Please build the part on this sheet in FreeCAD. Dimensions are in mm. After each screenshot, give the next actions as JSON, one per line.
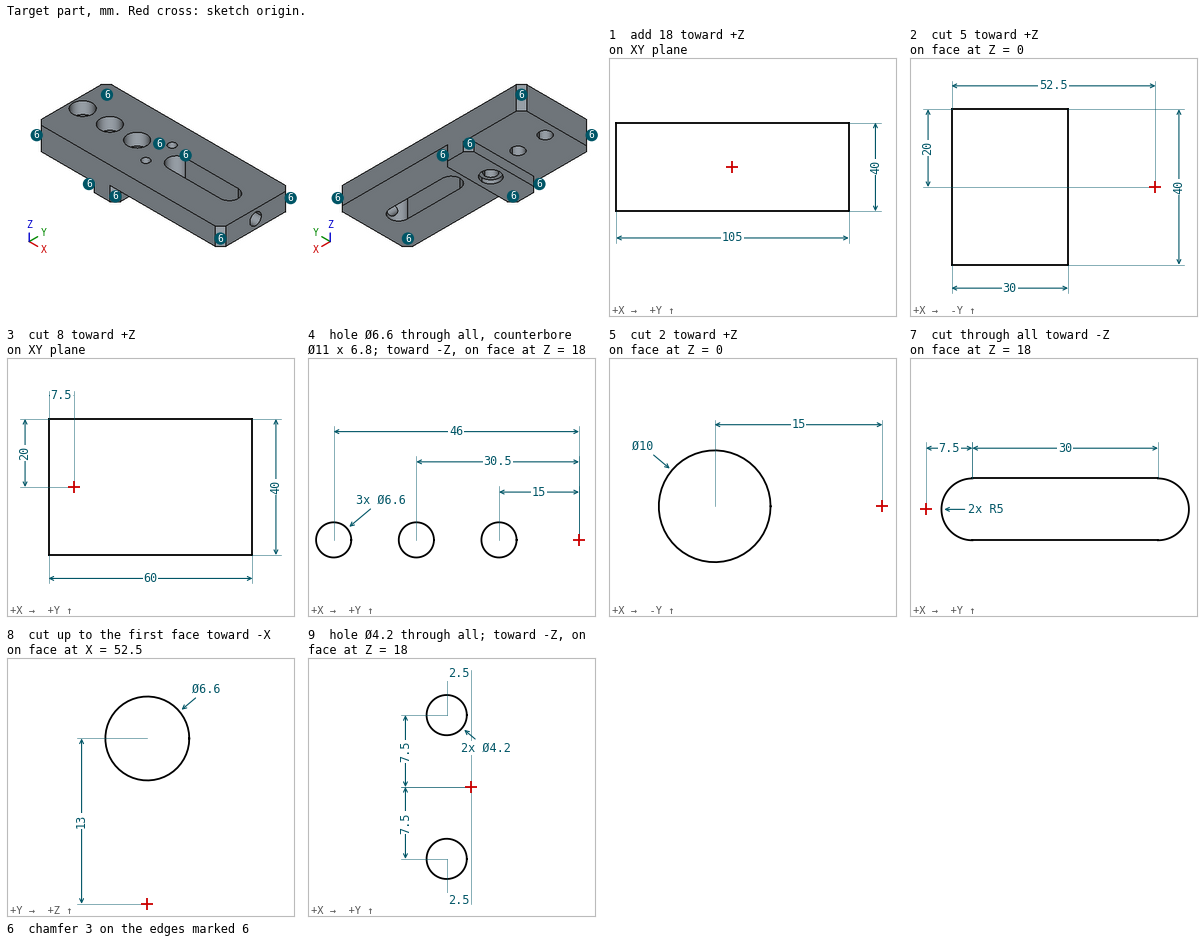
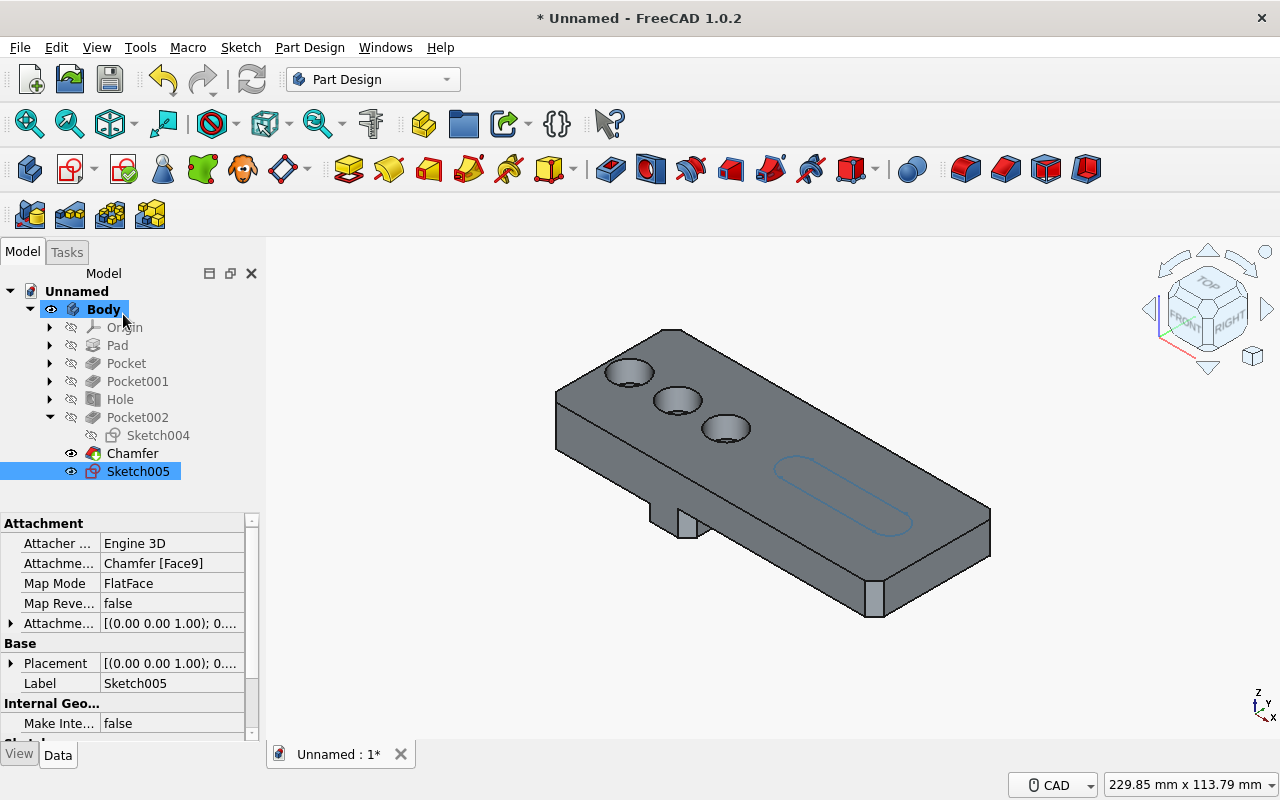
{"action": "left_click", "coordinate": [612, 170]}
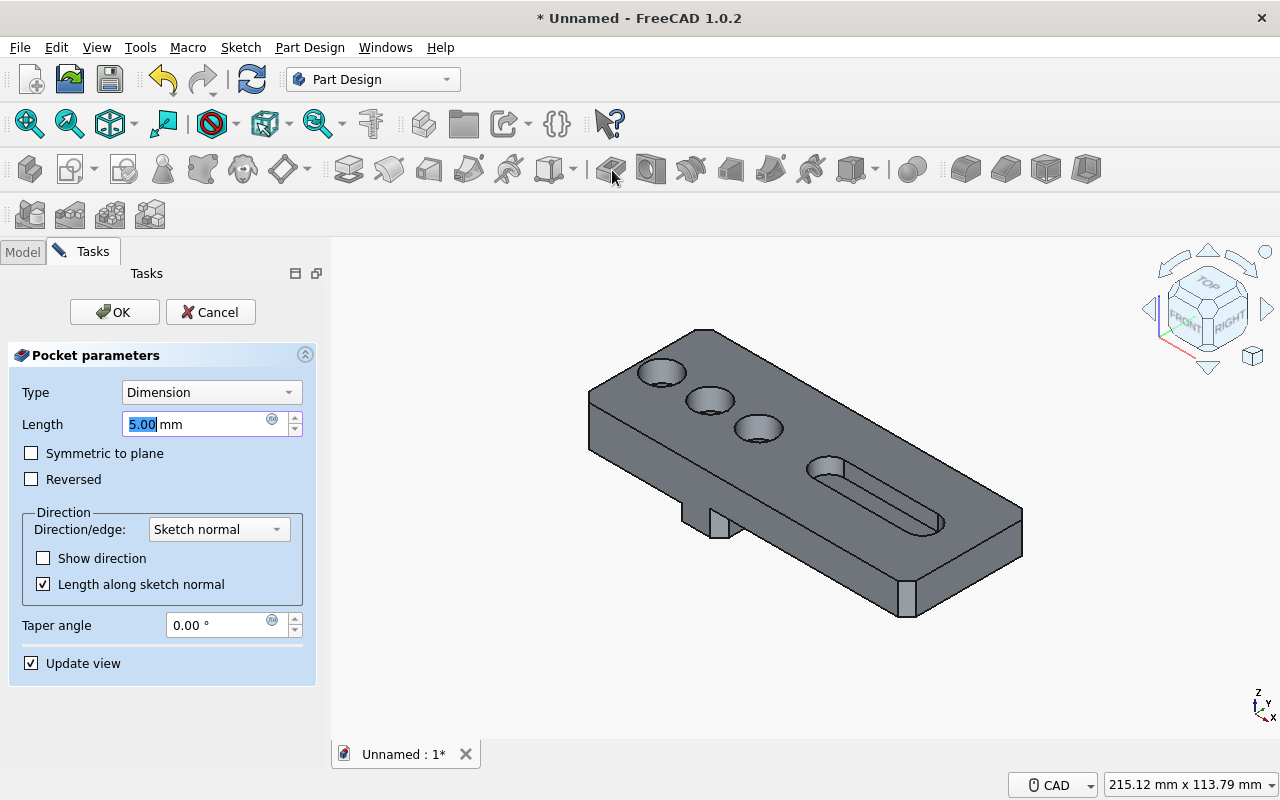
{"action": "left_click", "coordinate": [212, 392]}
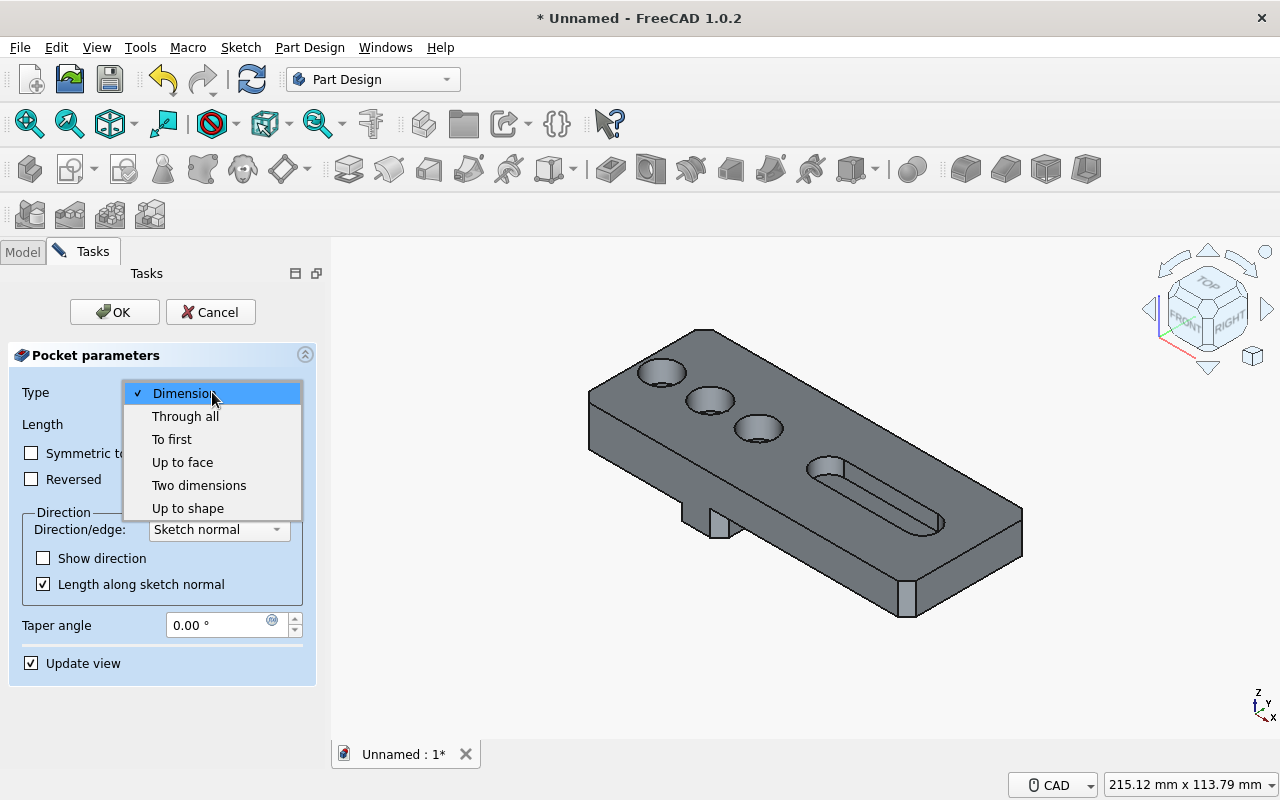
{"action": "left_click", "coordinate": [212, 416]}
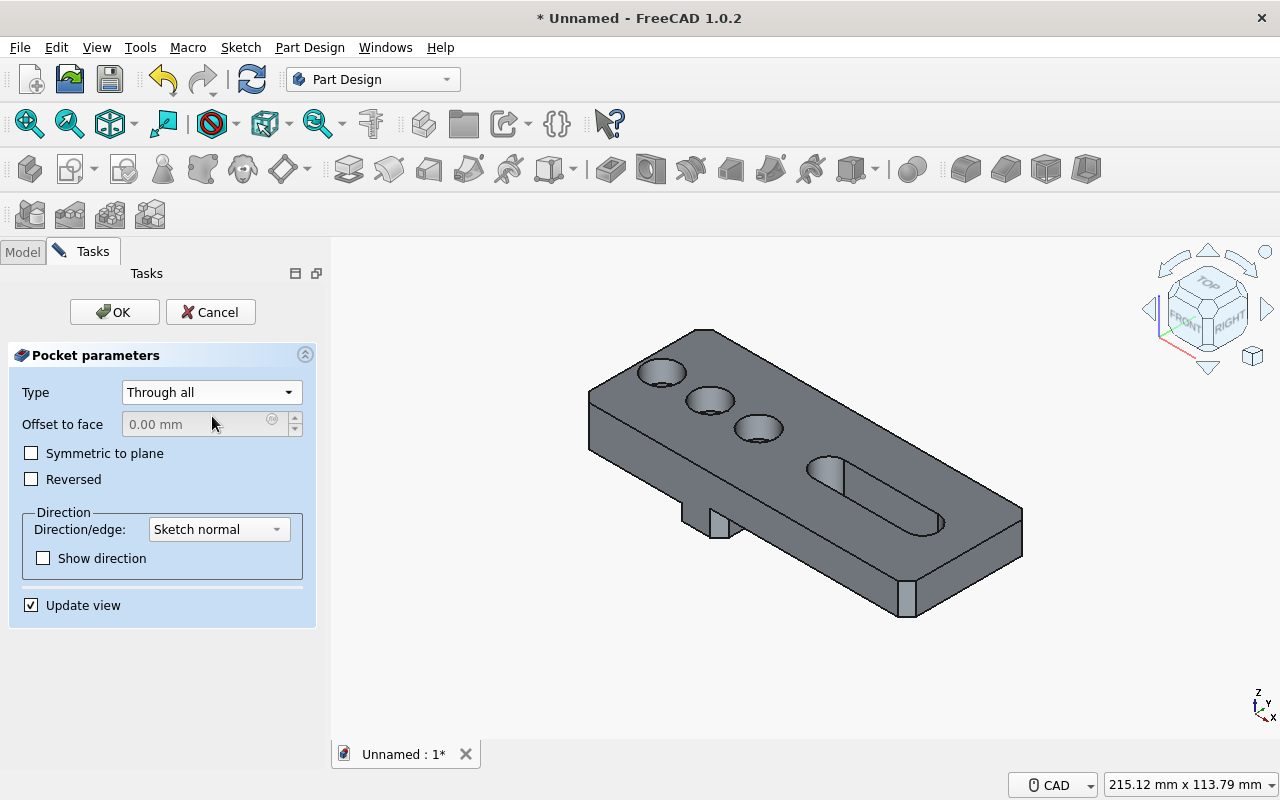
{"action": "left_click", "coordinate": [115, 312]}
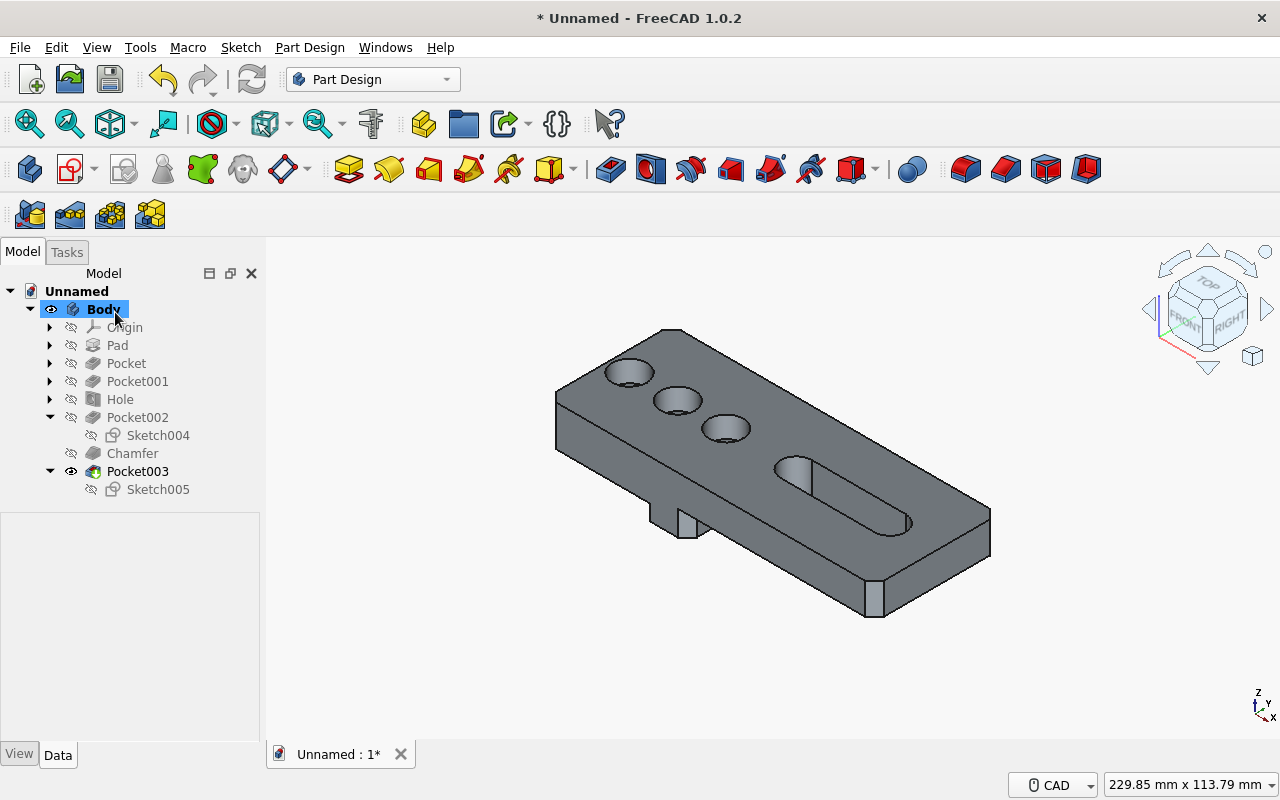
{"action": "left_click", "coordinate": [967, 550]}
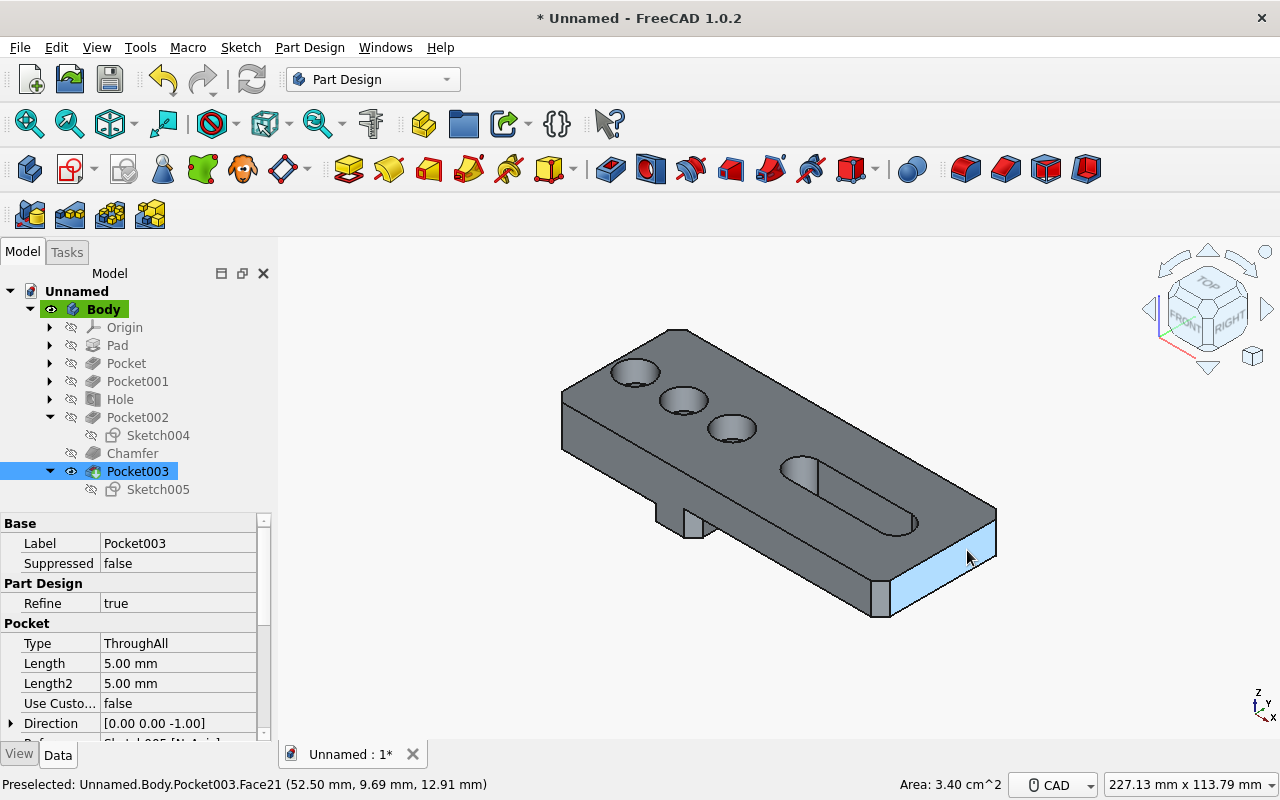
{"action": "left_click", "coordinate": [70, 170]}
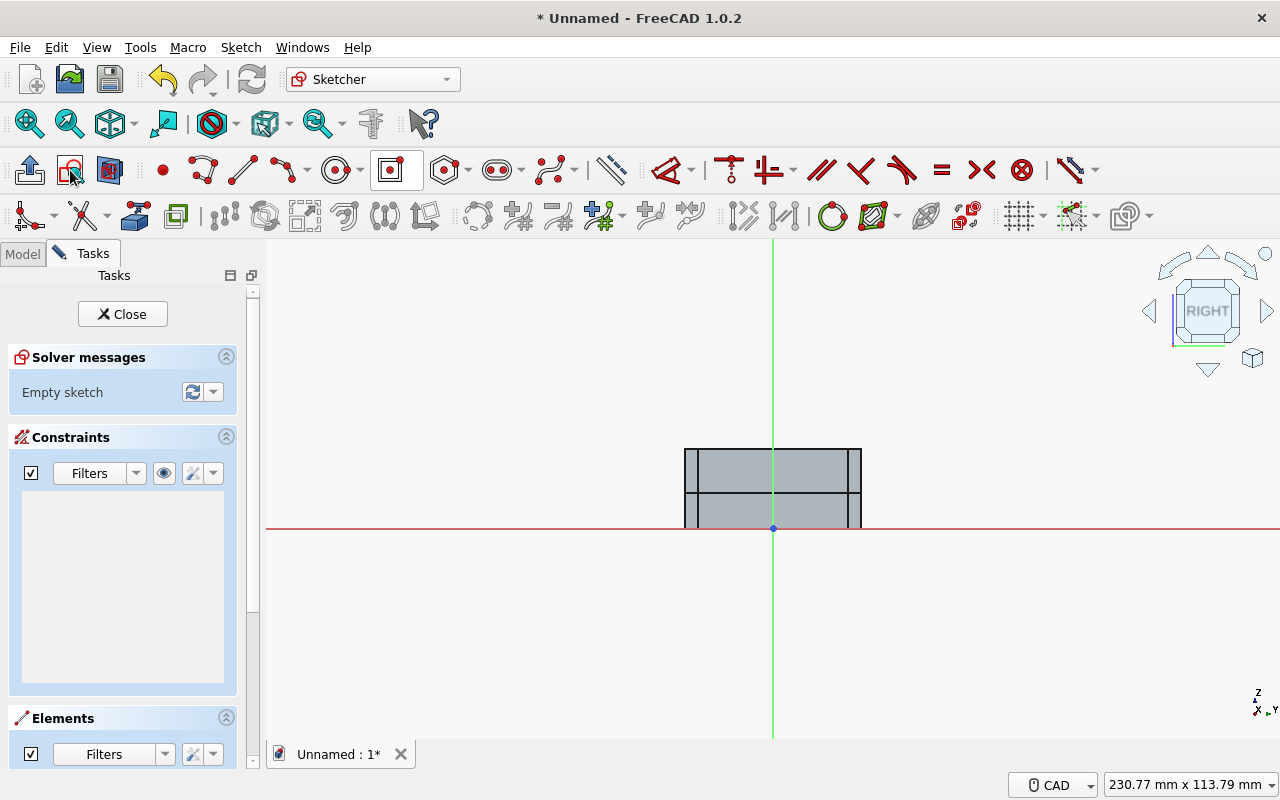
{"action": "scroll", "coordinate": [795, 494], "scroll_direction": "up", "scroll_amount": 7}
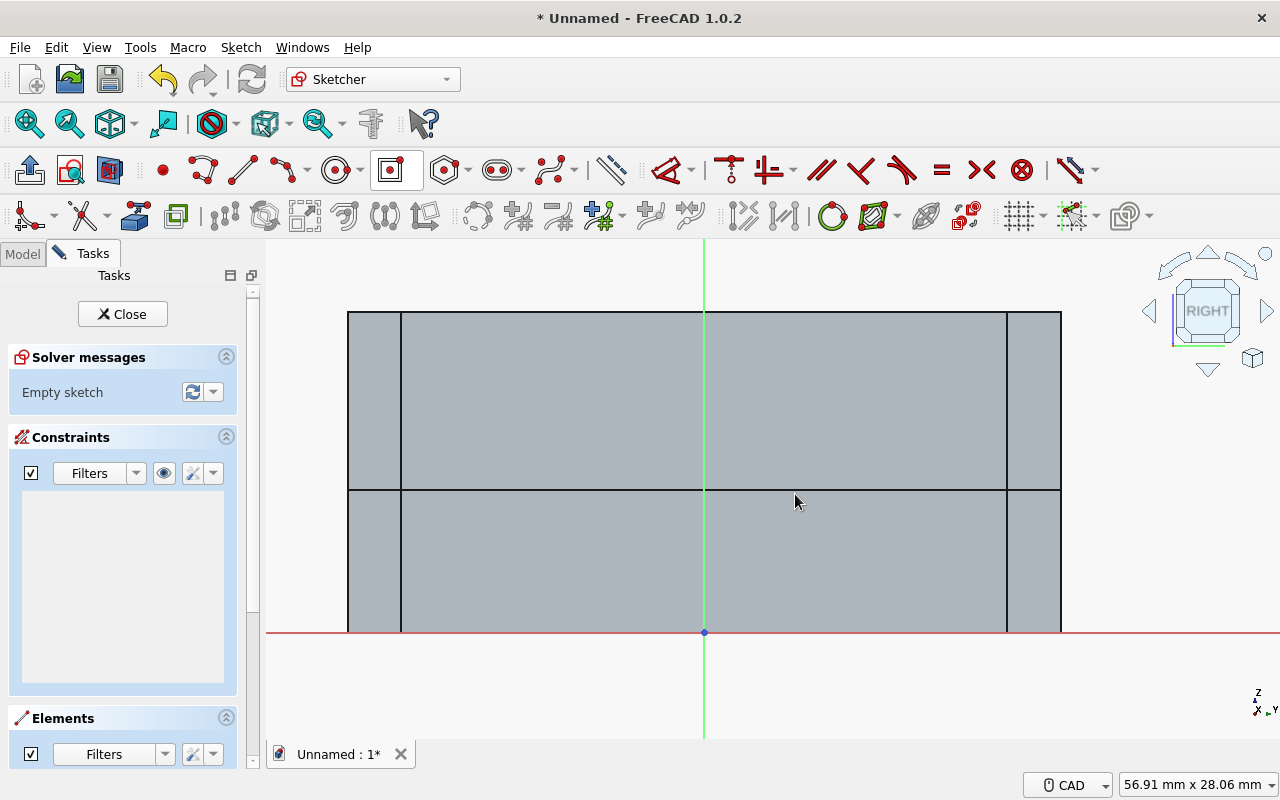
{"action": "left_click", "coordinate": [336, 170]}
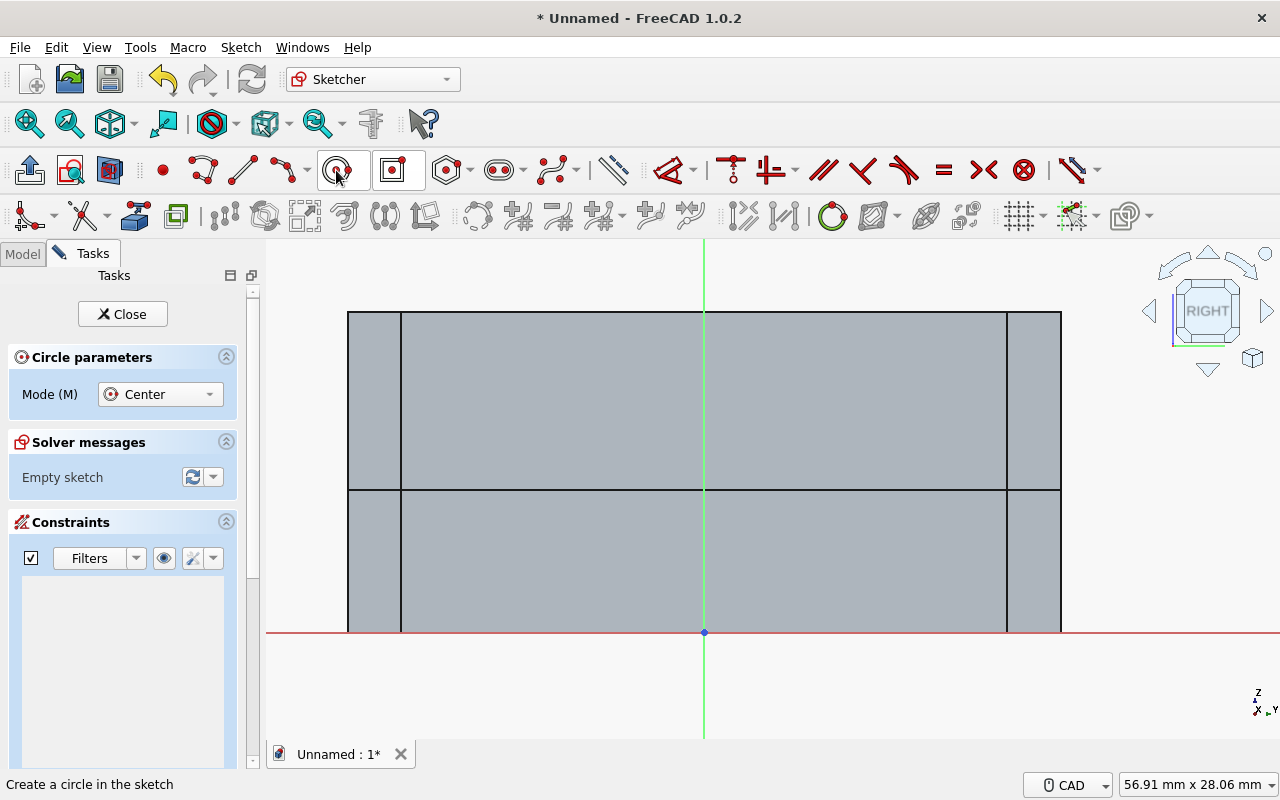
{"action": "left_click", "coordinate": [704, 401]}
{"action": "mouse_move", "coordinate": [746, 359]}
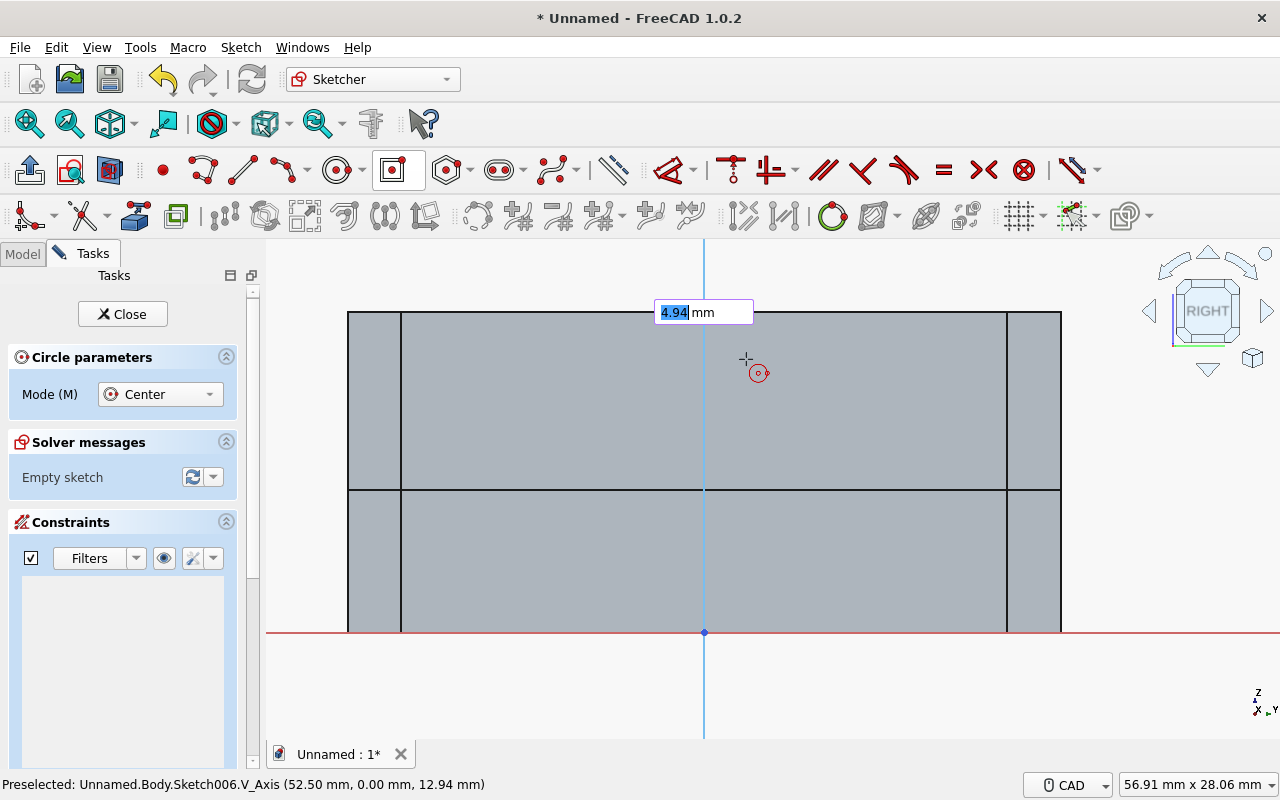
{"action": "type", "text": "6.6"}
{"action": "key", "text": "Return"}
{"action": "key", "text": "Escape"}